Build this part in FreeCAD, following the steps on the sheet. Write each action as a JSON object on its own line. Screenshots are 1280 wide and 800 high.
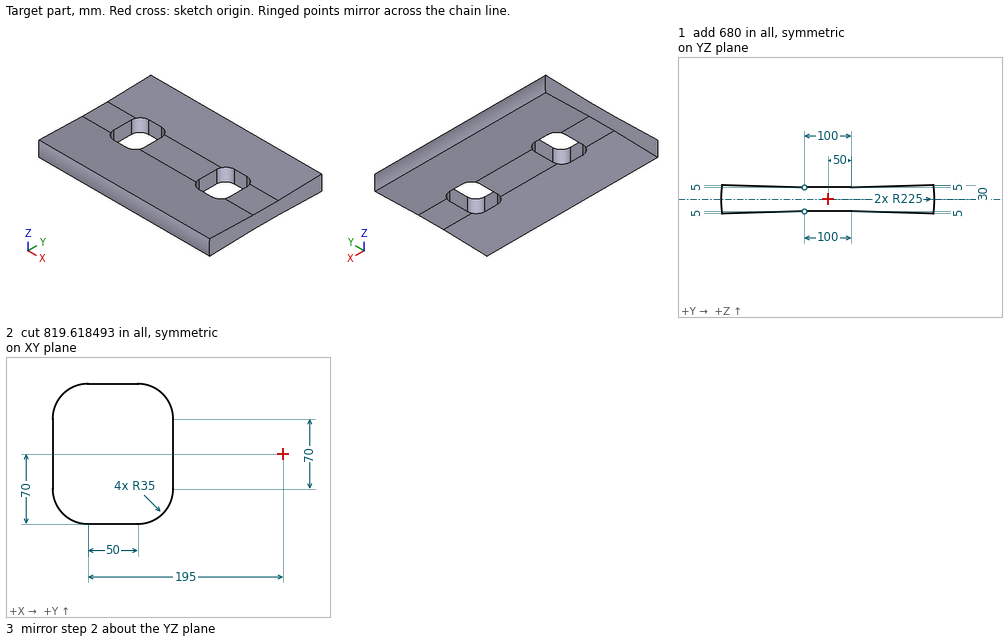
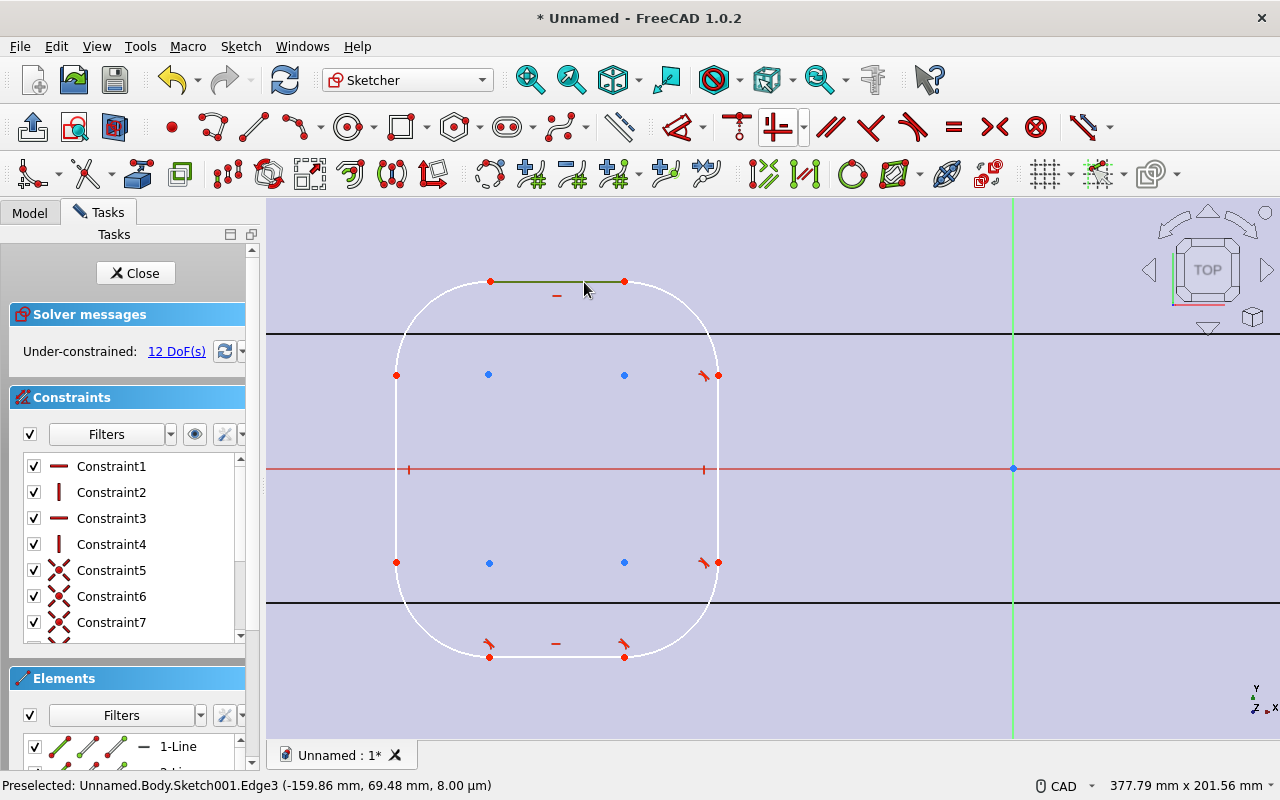
{"action": "left_click", "coordinate": [708, 333]}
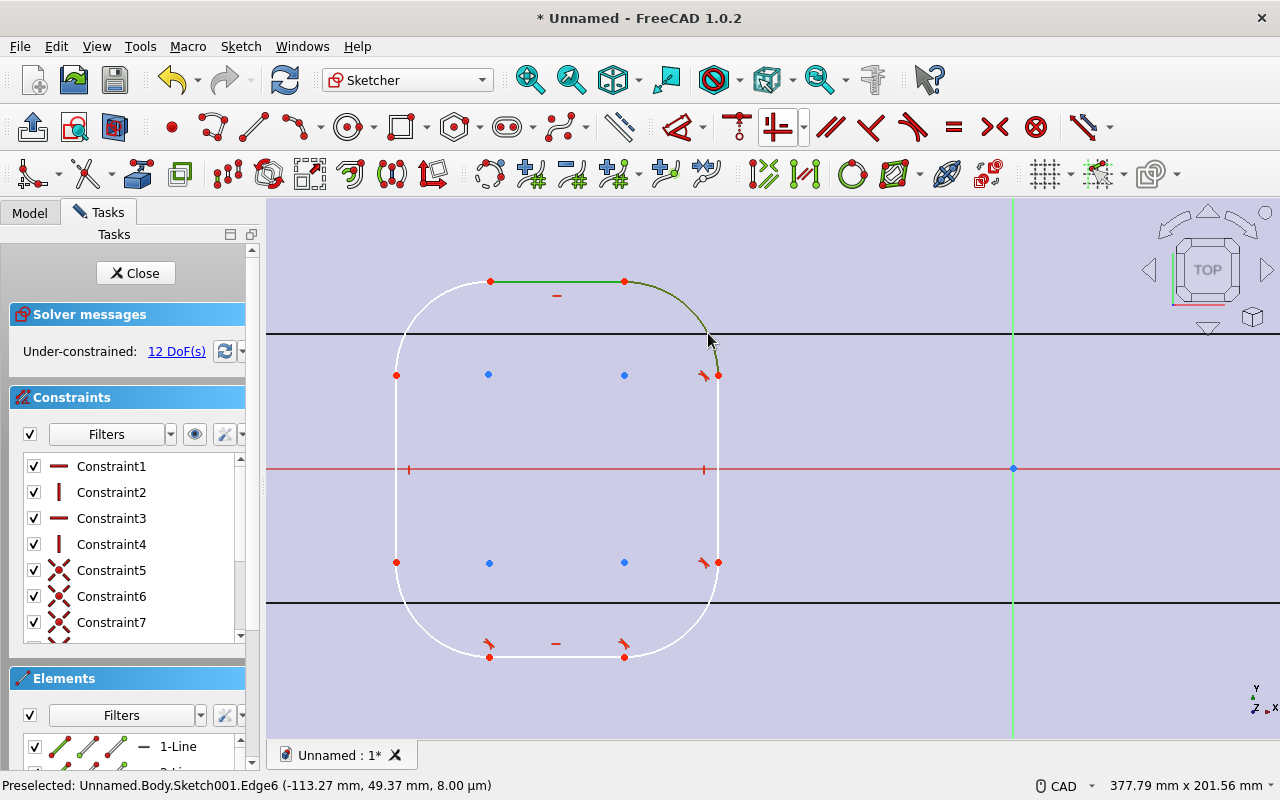
{"action": "left_click", "coordinate": [913, 128]}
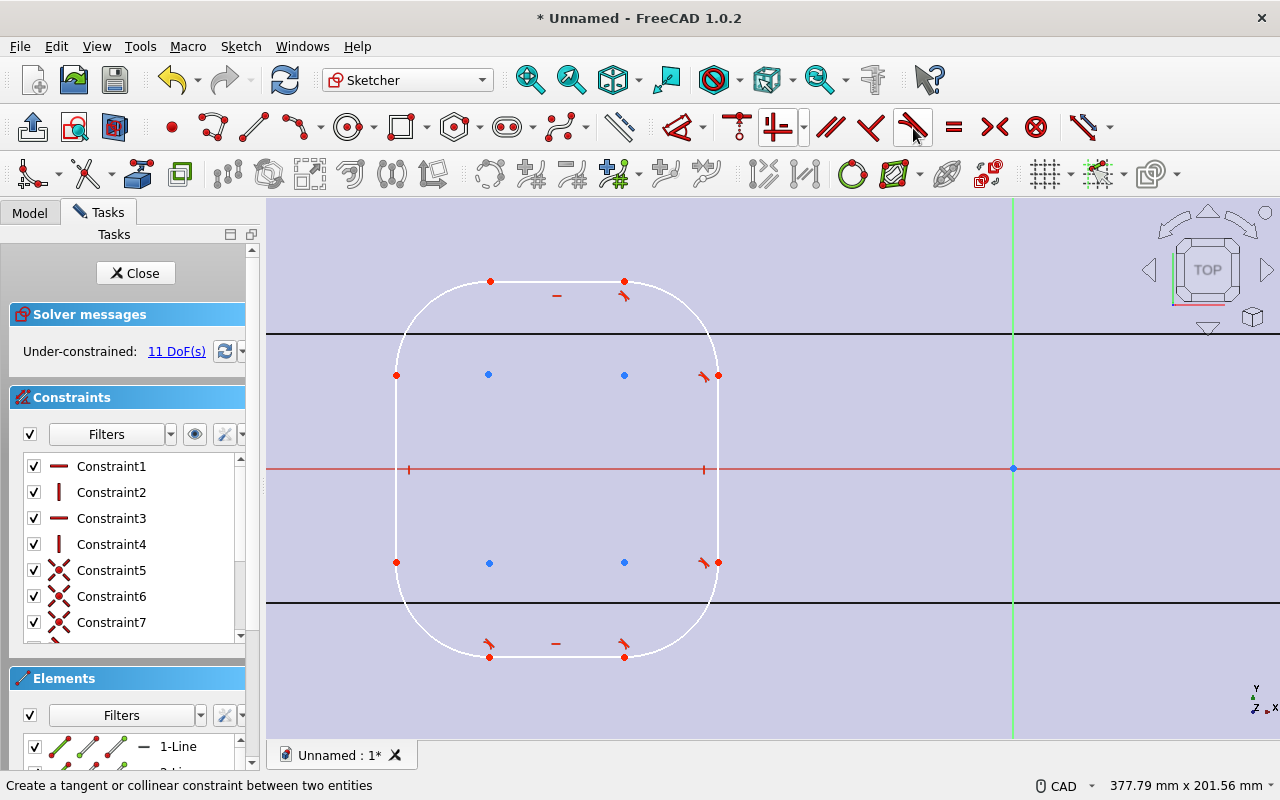
{"action": "left_click", "coordinate": [584, 282]}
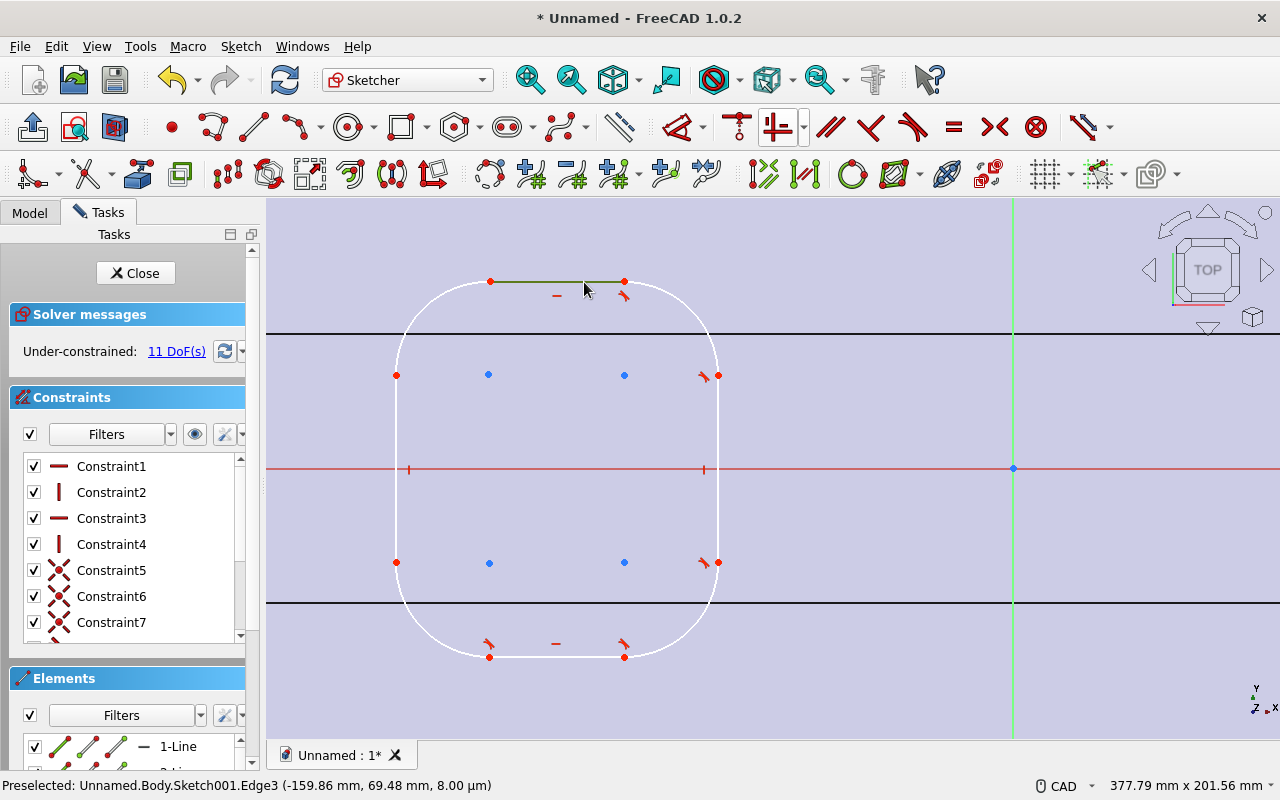
{"action": "left_click", "coordinate": [447, 292]}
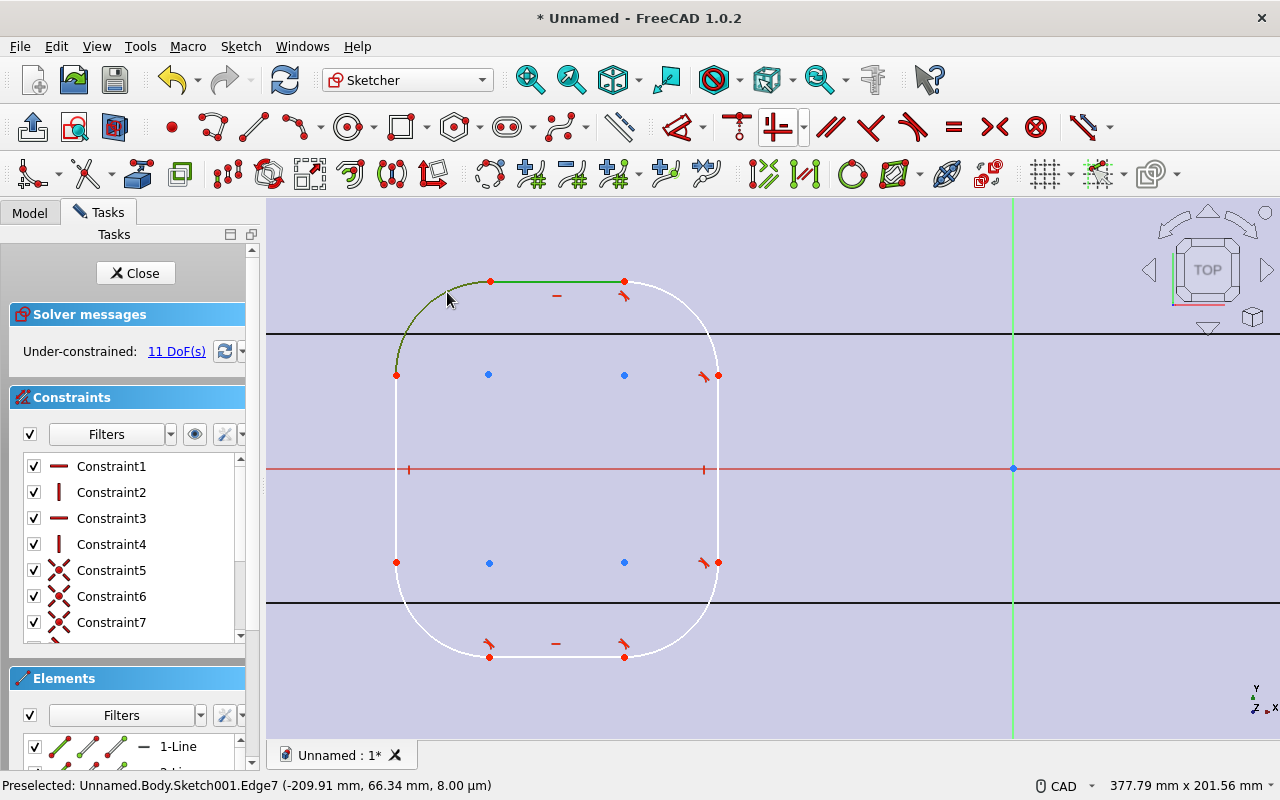
{"action": "key", "text": "t"}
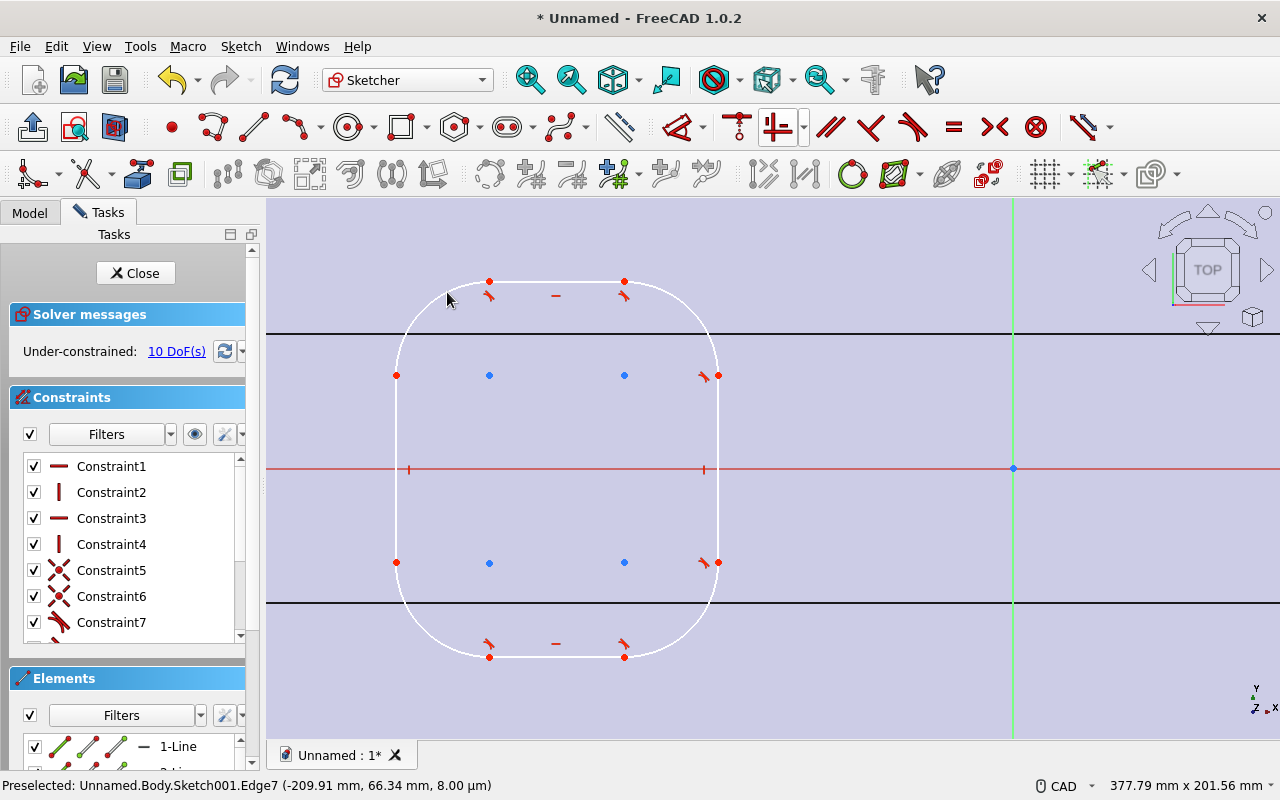
{"action": "left_click", "coordinate": [396, 432]}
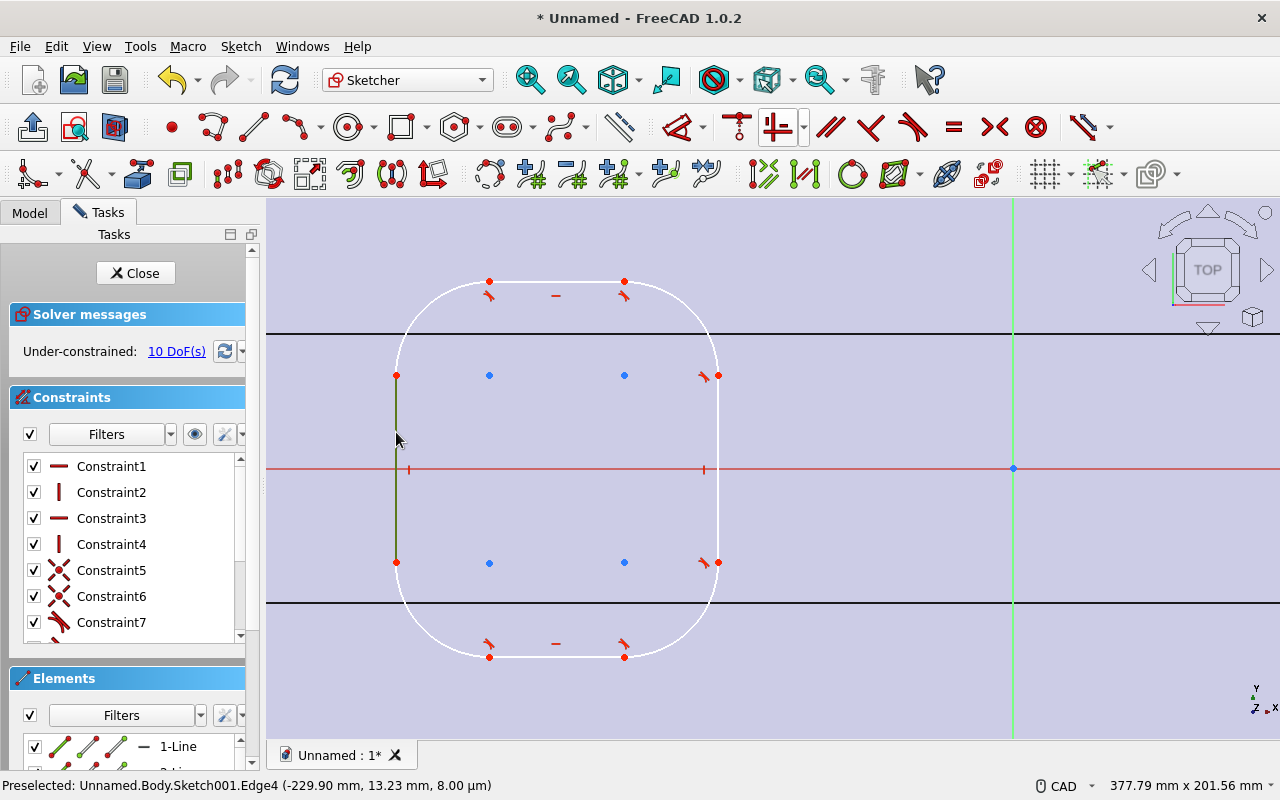
{"action": "left_click", "coordinate": [447, 292]}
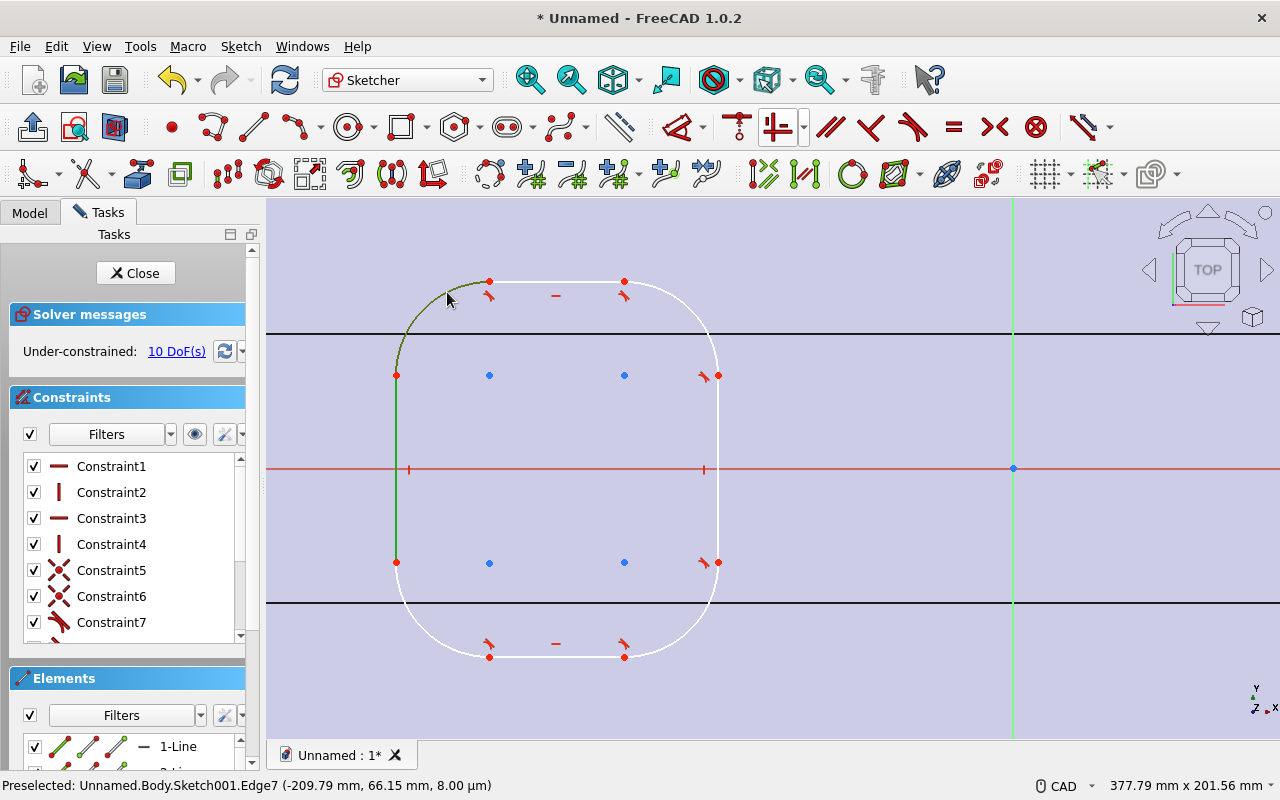
{"action": "key", "text": "t"}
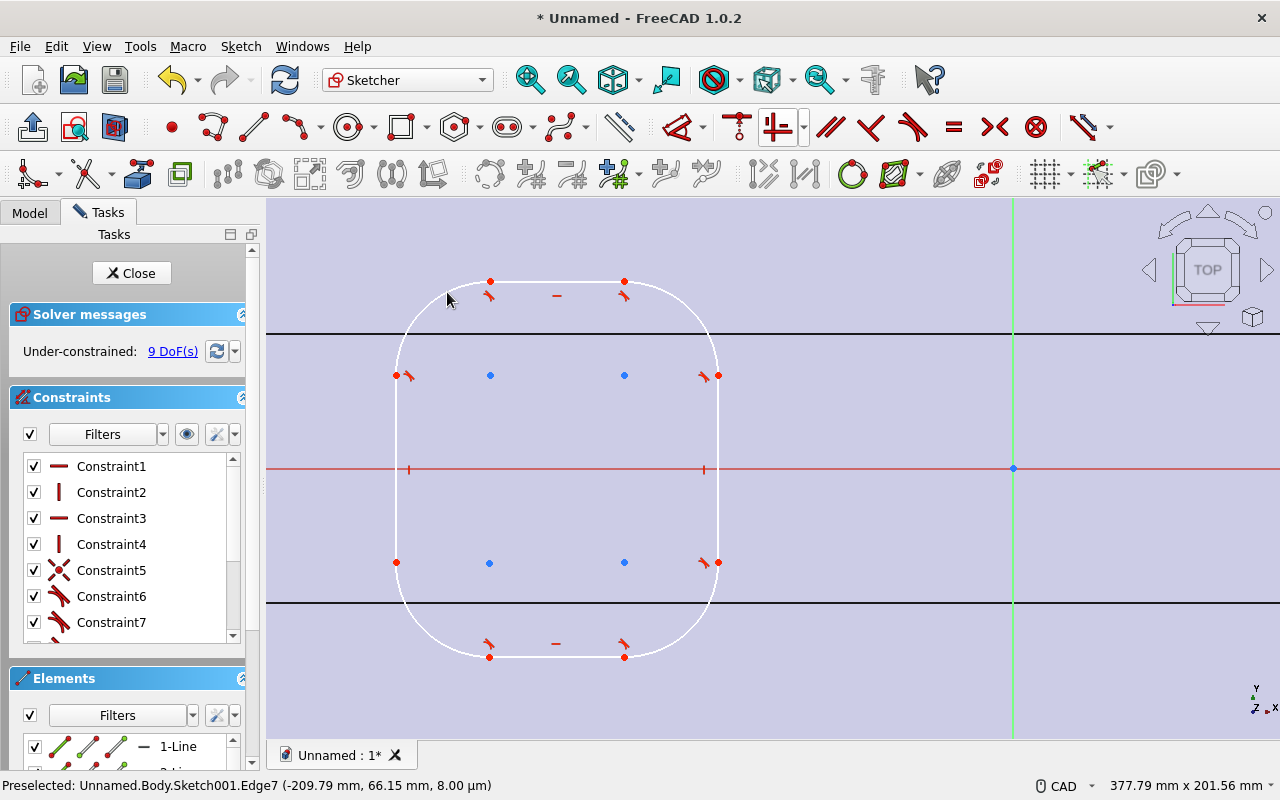
{"action": "left_click", "coordinate": [396, 432]}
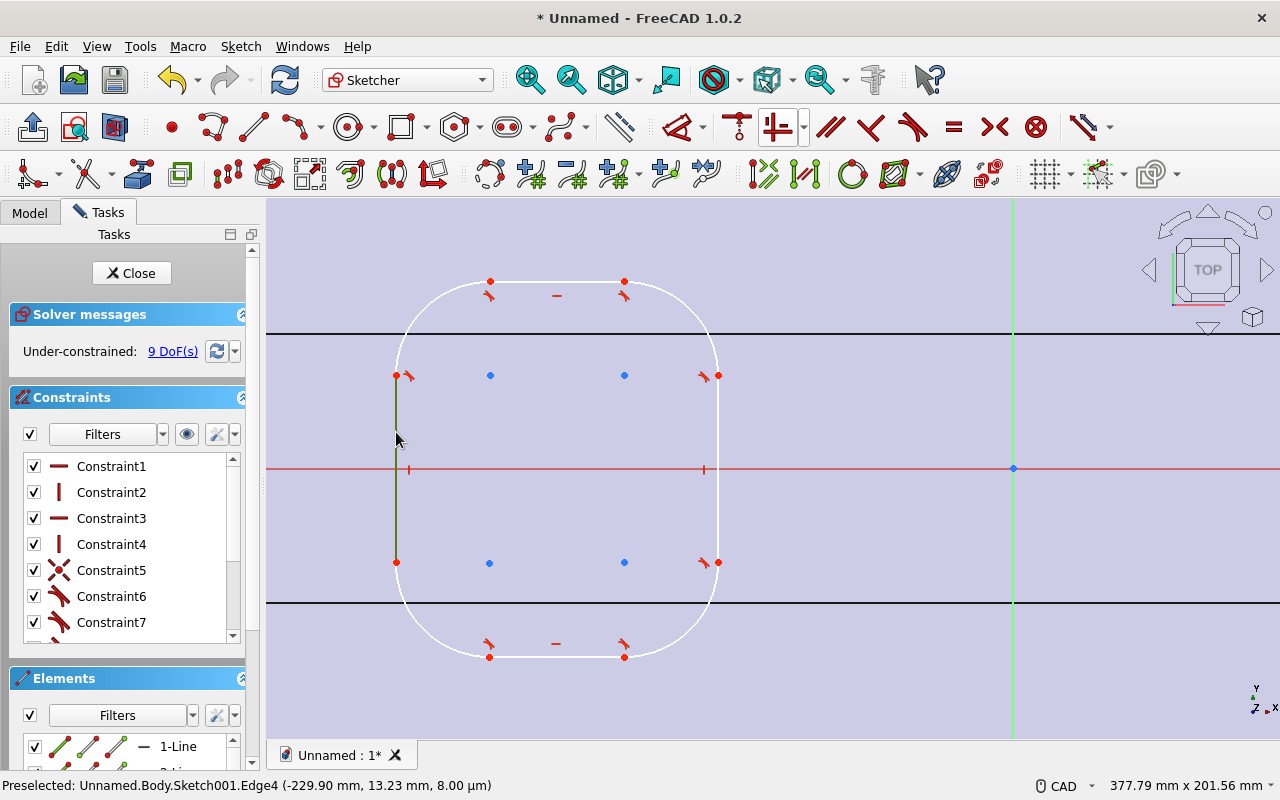
{"action": "left_click", "coordinate": [406, 606]}